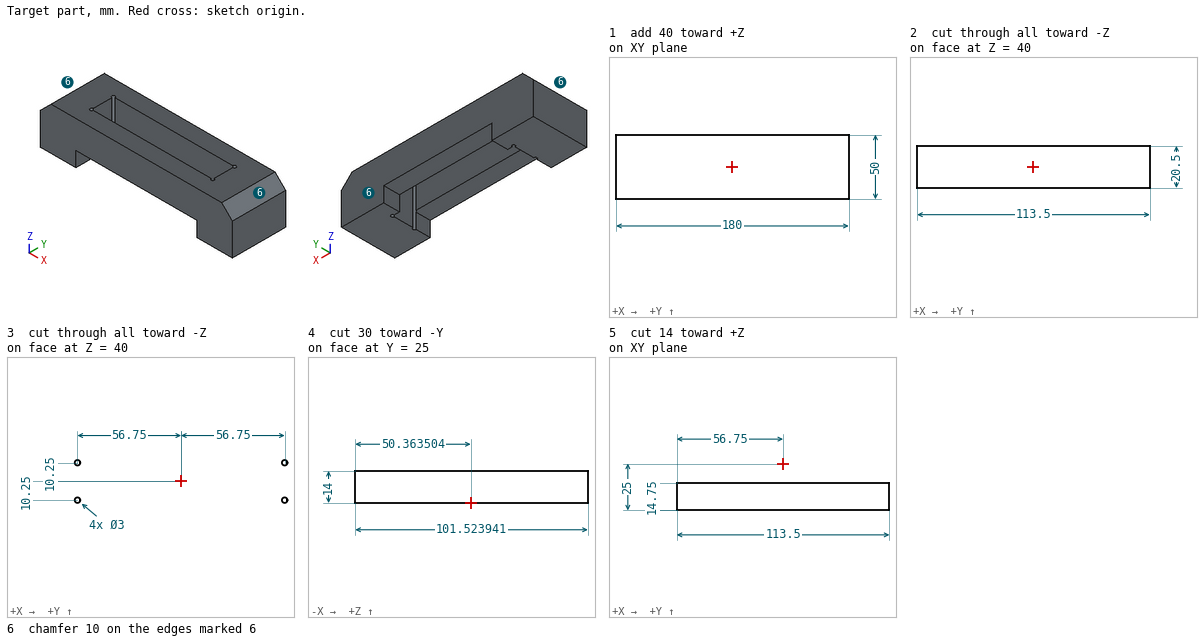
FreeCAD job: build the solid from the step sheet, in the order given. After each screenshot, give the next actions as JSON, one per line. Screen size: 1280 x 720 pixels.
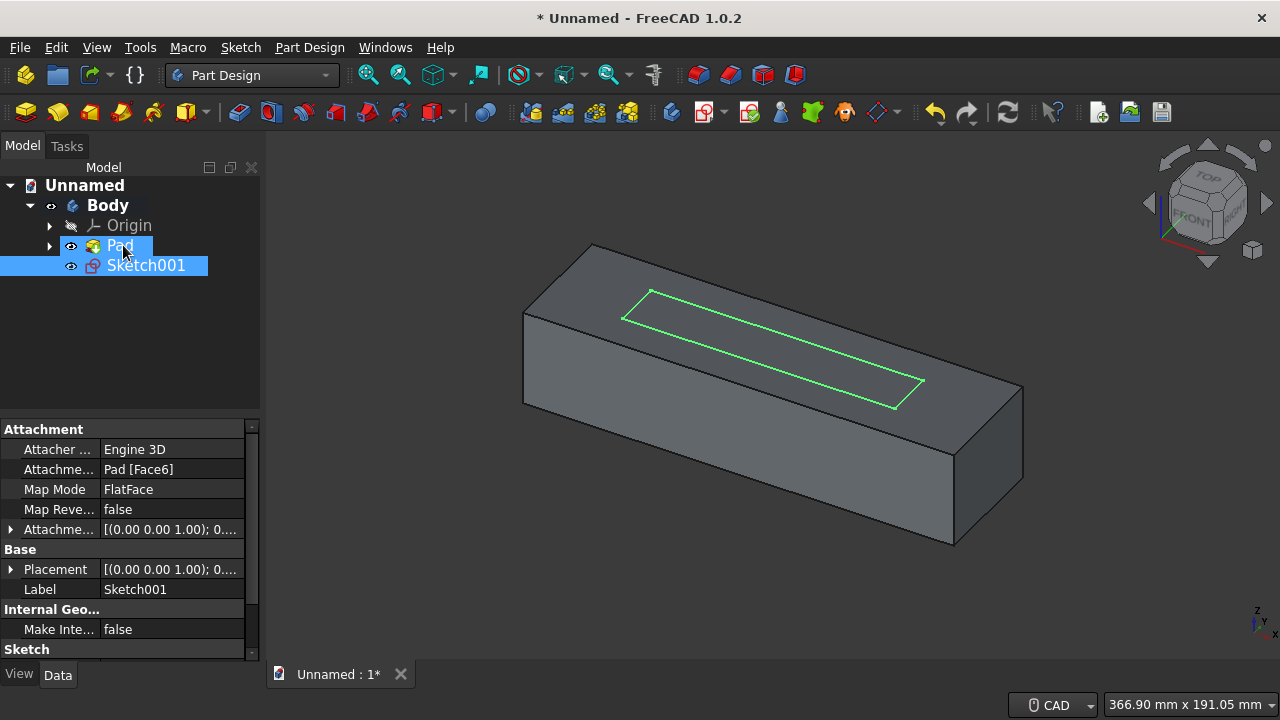
{"action": "left_click", "coordinate": [240, 112]}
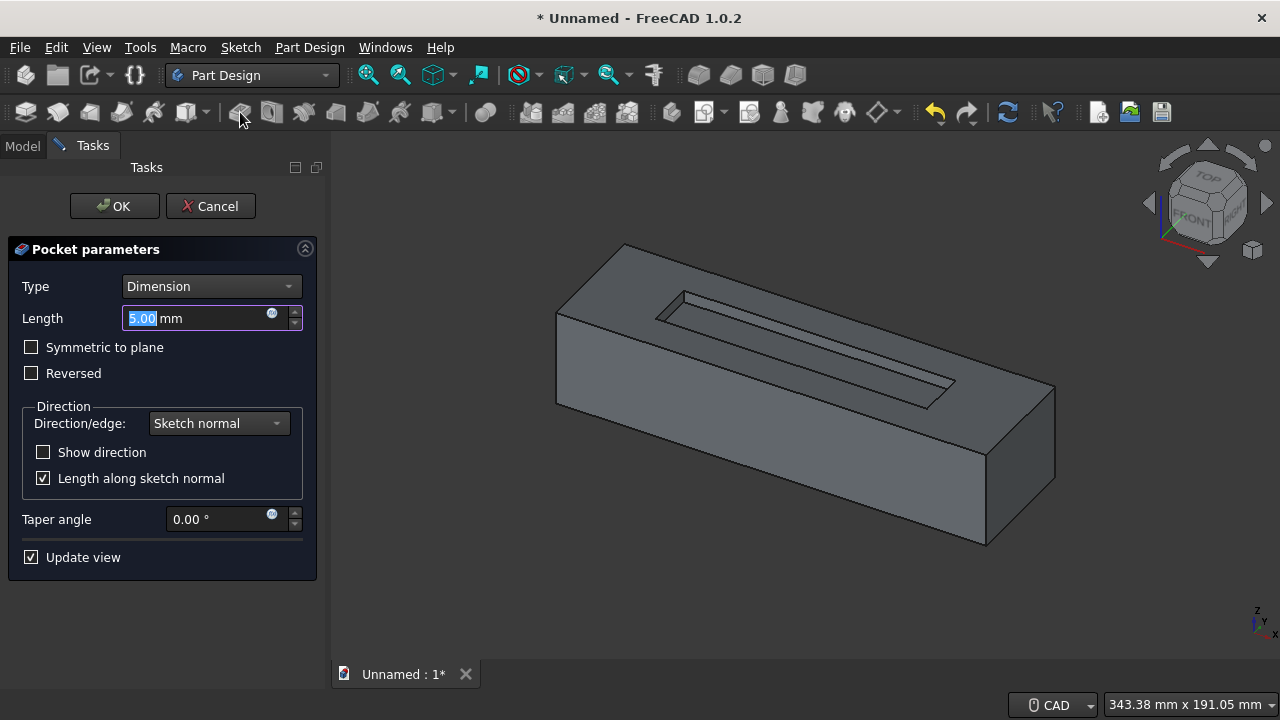
{"action": "left_click", "coordinate": [212, 286]}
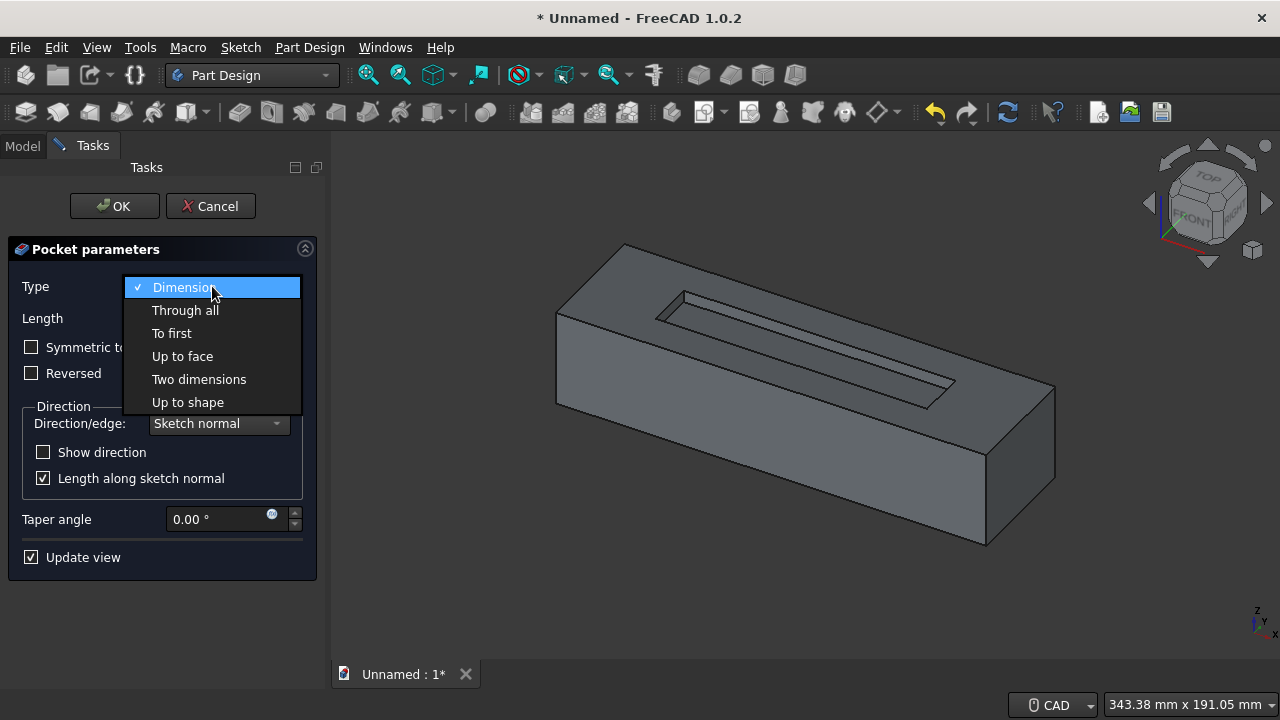
{"action": "left_click", "coordinate": [212, 310]}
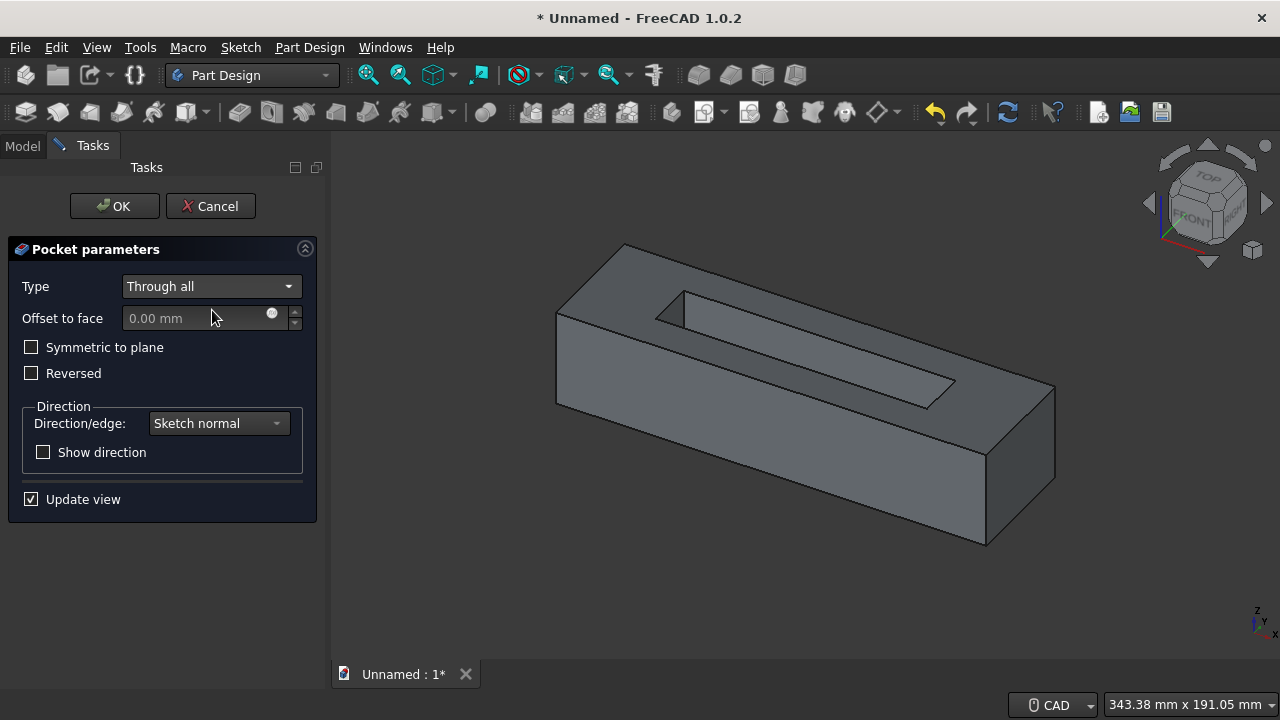
{"action": "left_click", "coordinate": [115, 206]}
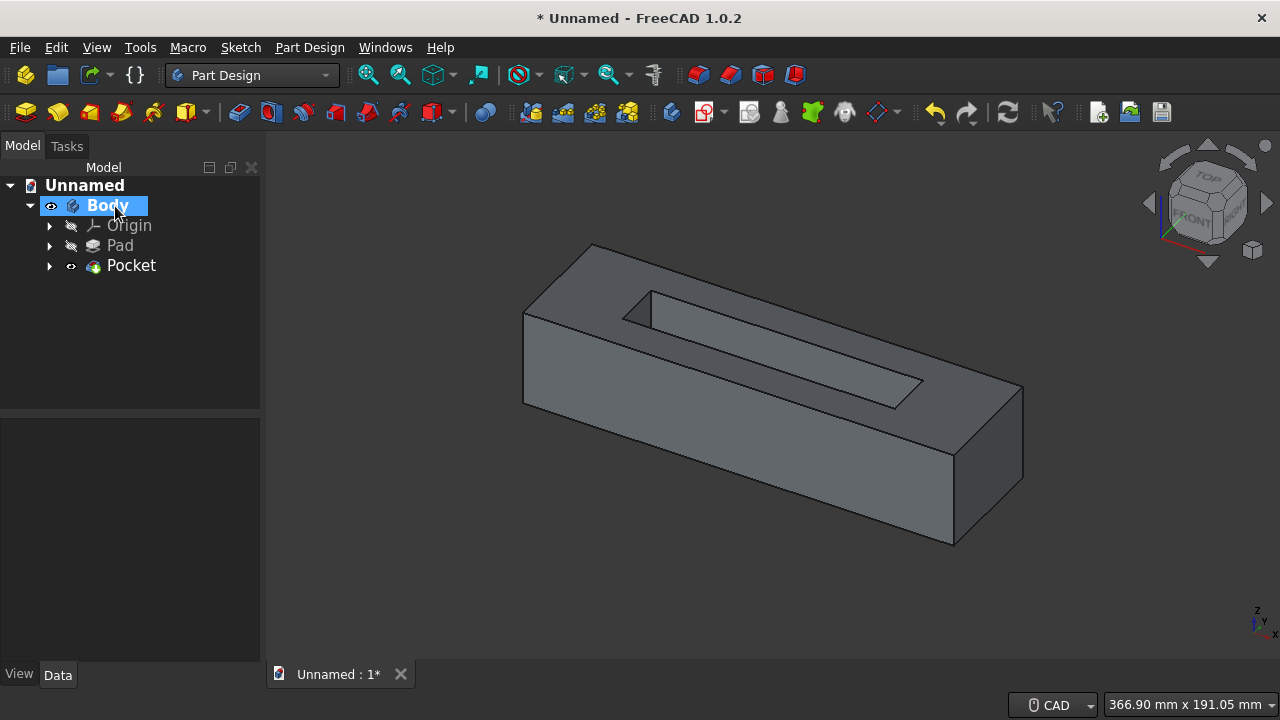
{"action": "left_click", "coordinate": [968, 400]}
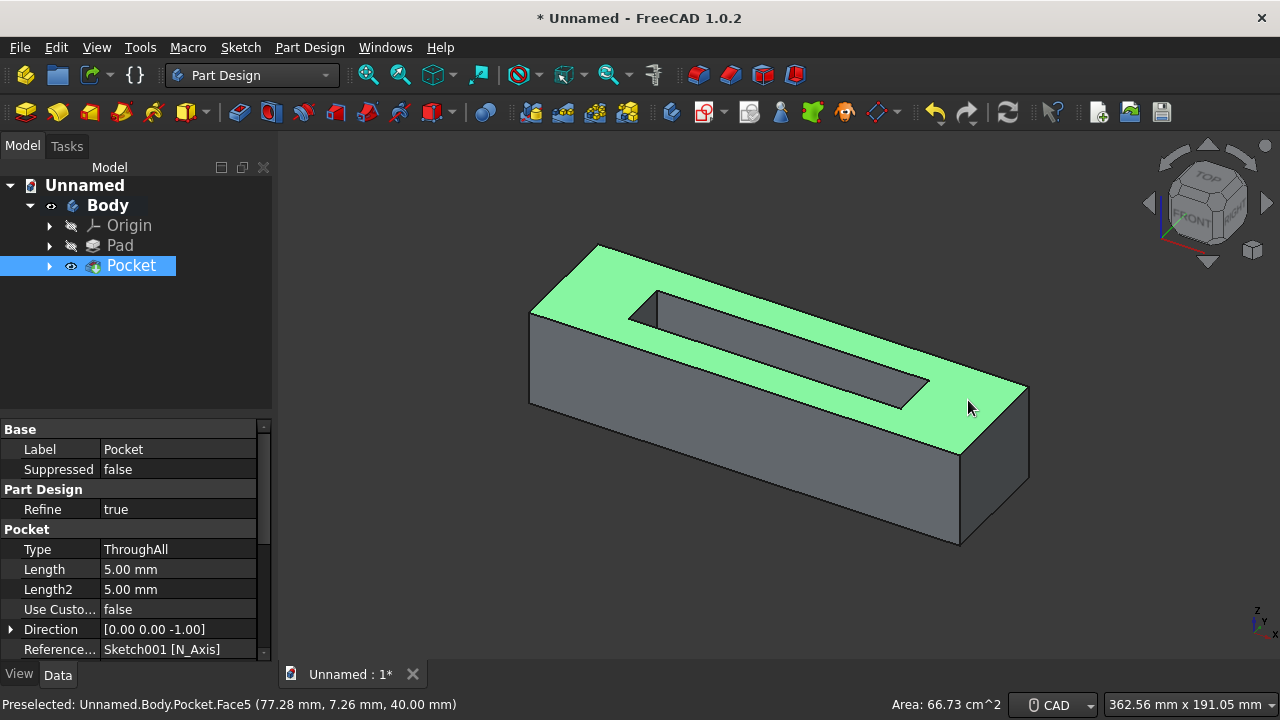
{"action": "left_click", "coordinate": [704, 112]}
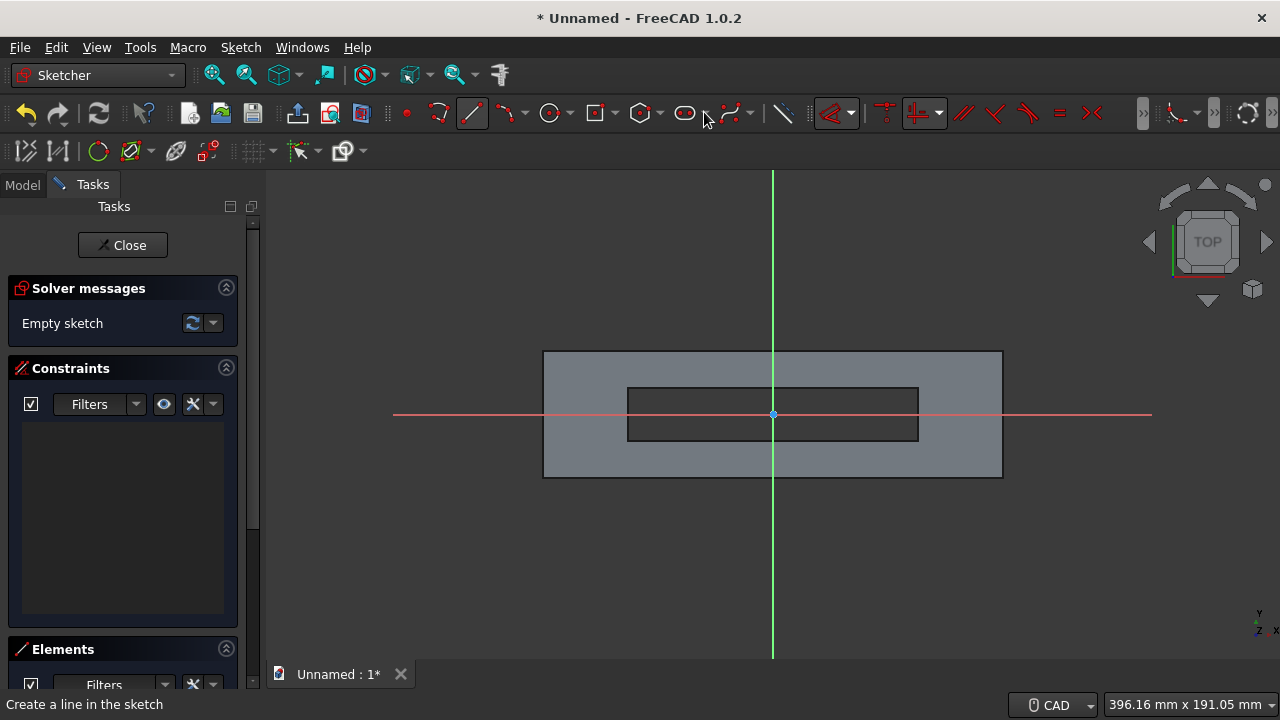
{"action": "scroll", "coordinate": [856, 415], "scroll_direction": "up", "scroll_amount": 3}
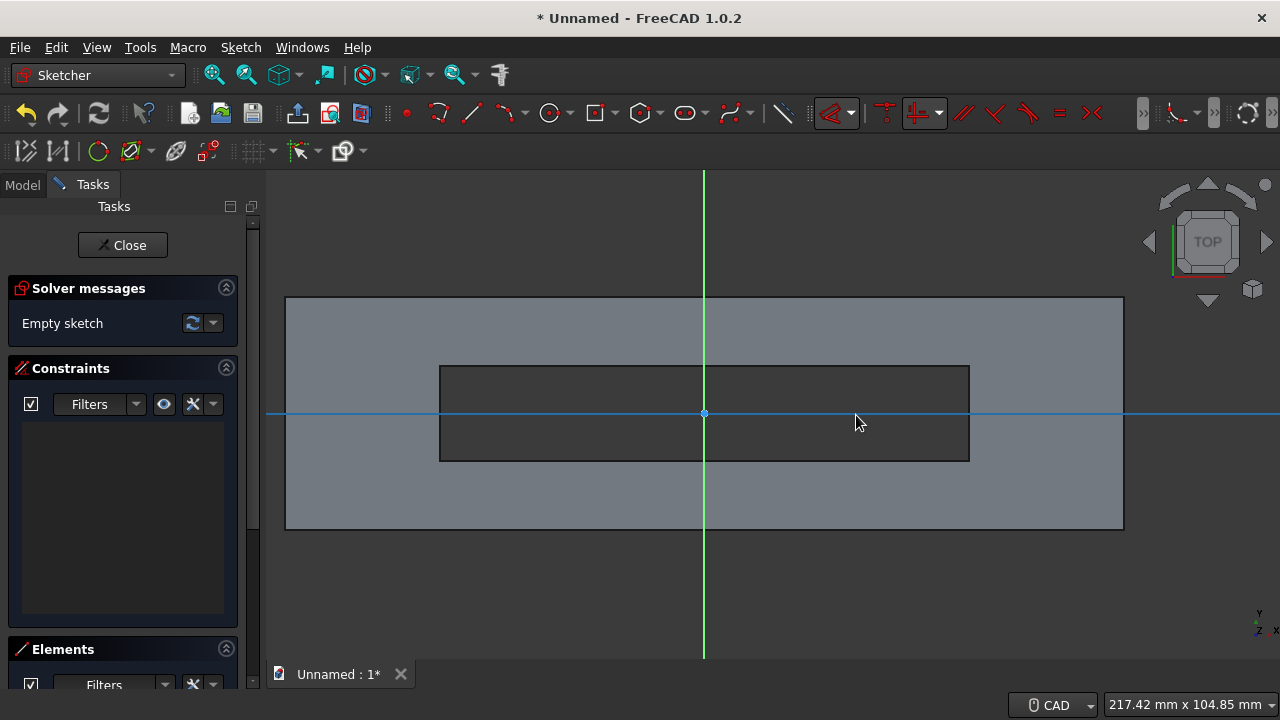
{"action": "left_click", "coordinate": [550, 114]}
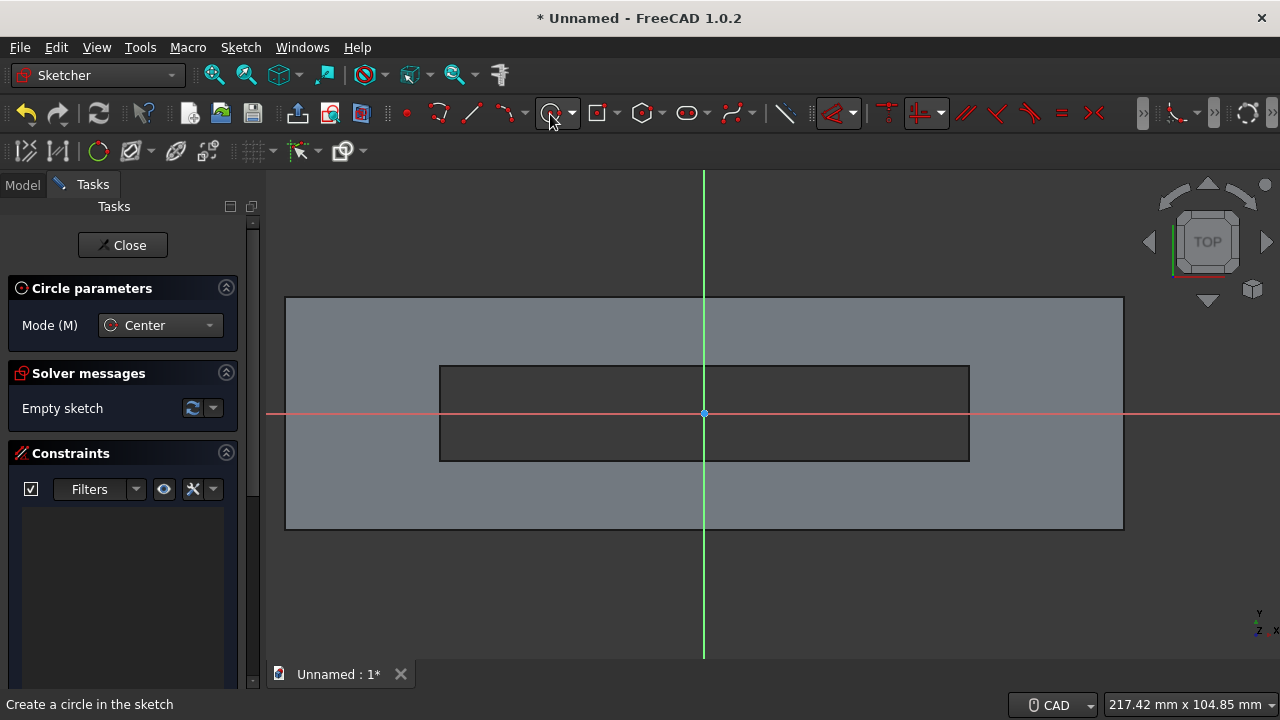
{"action": "scroll", "coordinate": [440, 366], "scroll_direction": "up", "scroll_amount": 6}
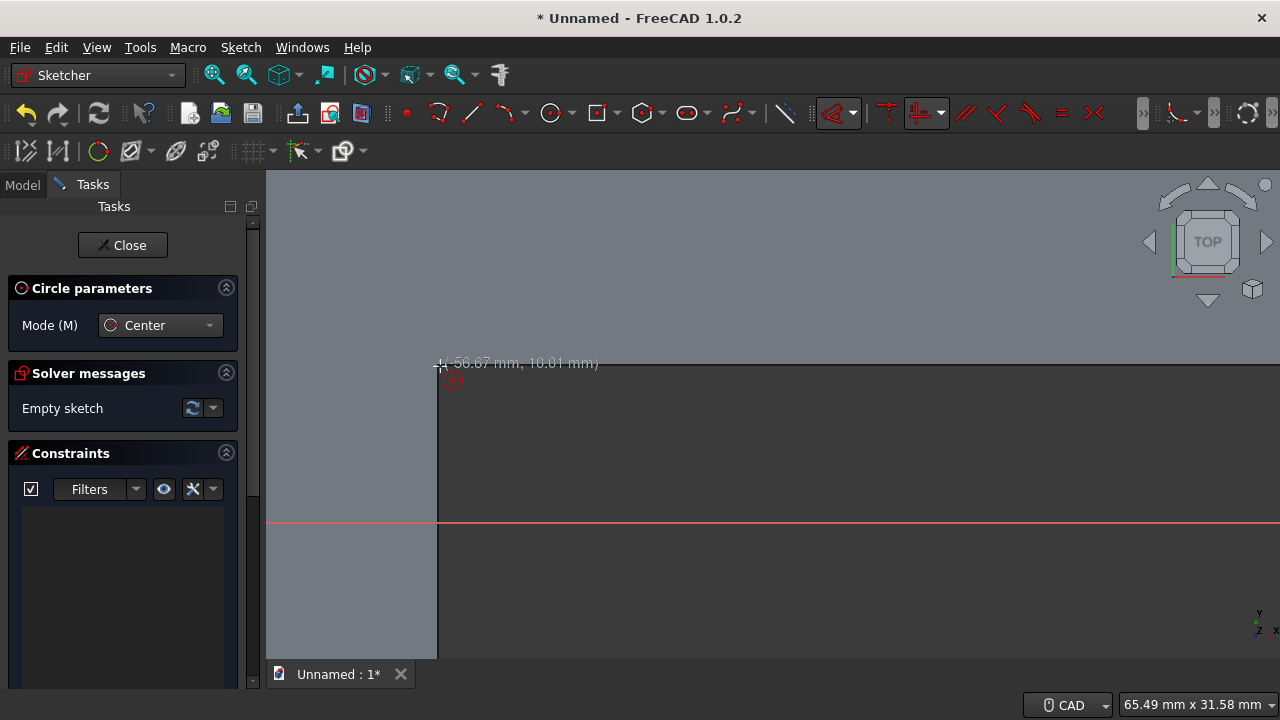
{"action": "left_click", "coordinate": [438, 365]}
{"action": "left_click", "coordinate": [455, 348]}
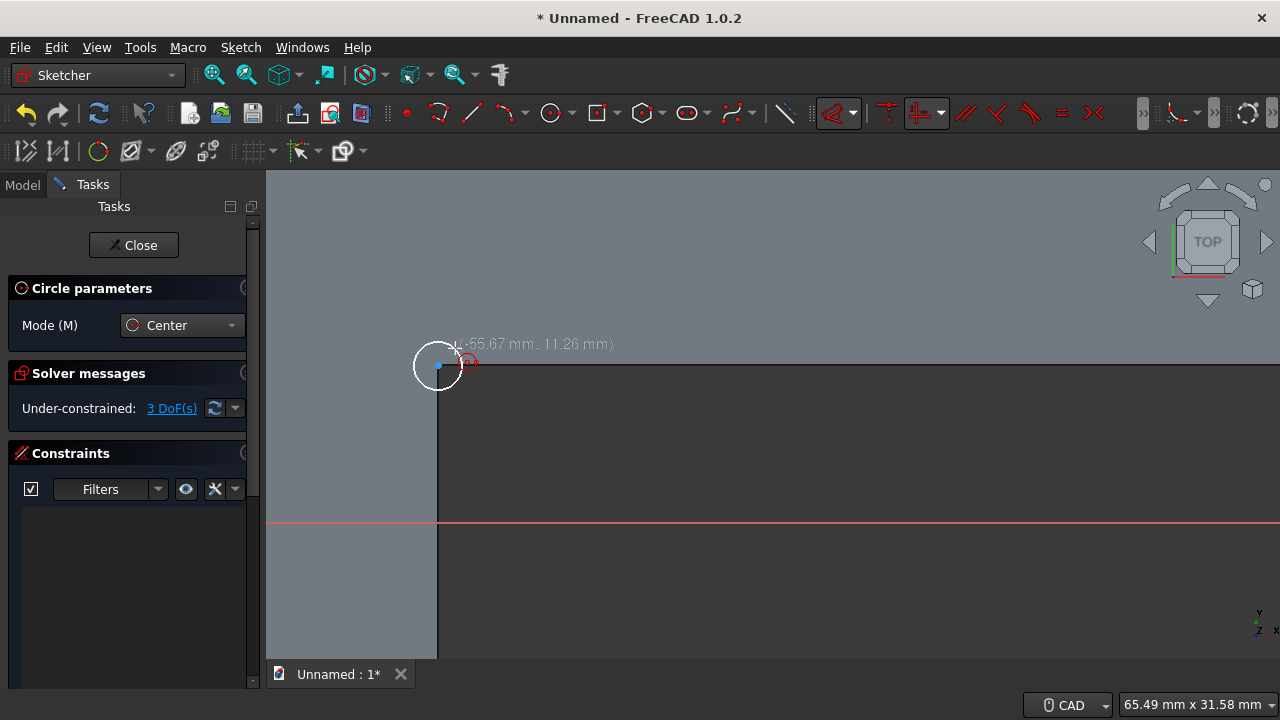
{"action": "scroll", "coordinate": [440, 368], "scroll_direction": "down", "scroll_amount": 6}